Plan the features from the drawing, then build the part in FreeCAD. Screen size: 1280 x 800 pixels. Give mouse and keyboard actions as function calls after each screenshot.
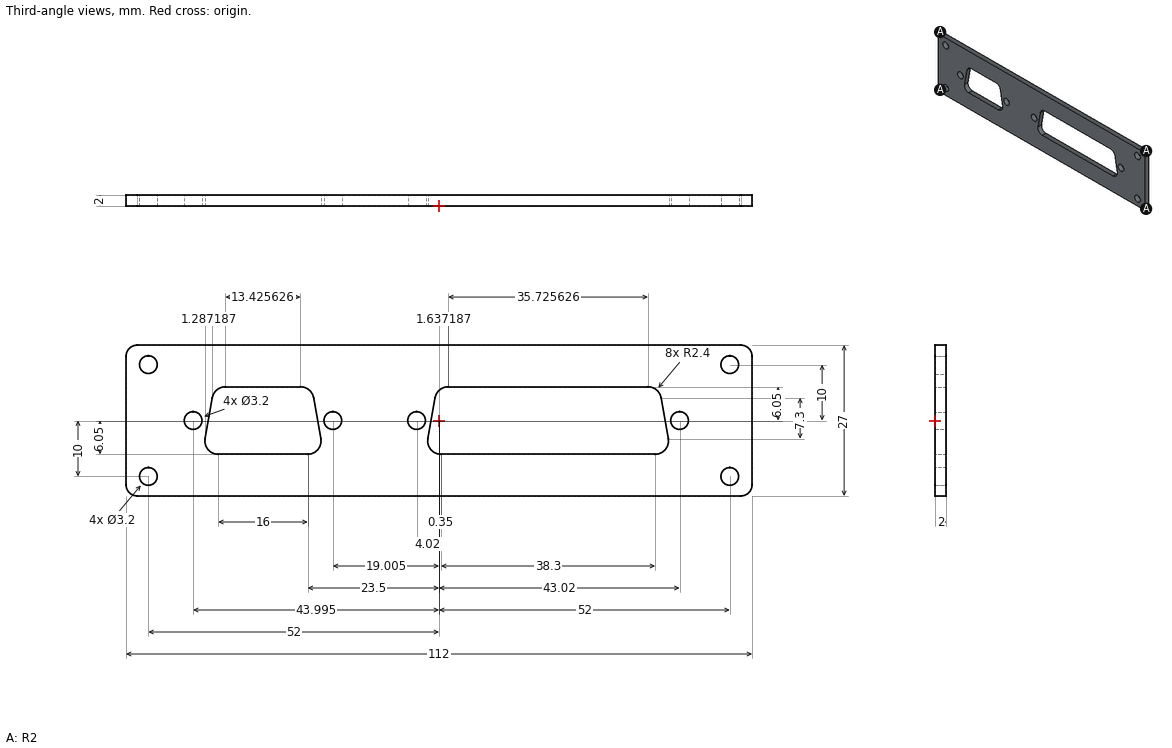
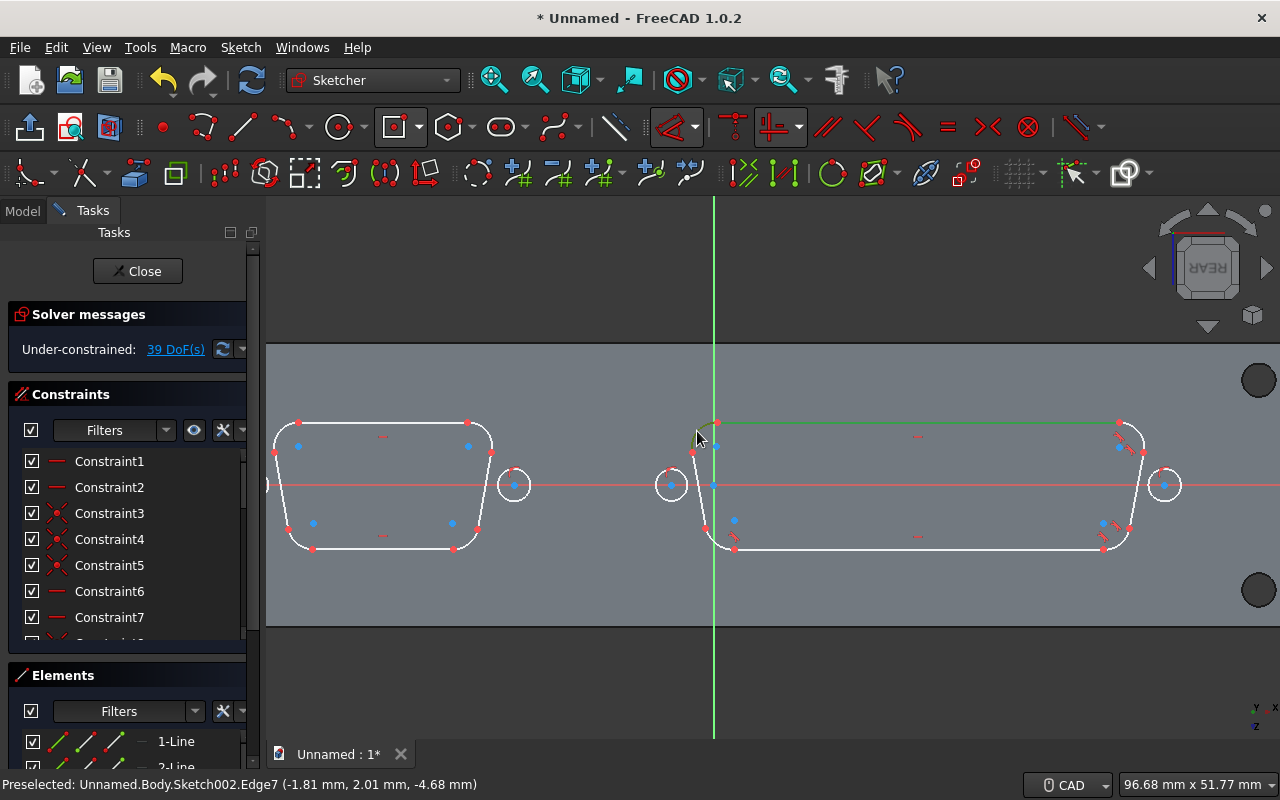
click(908, 128)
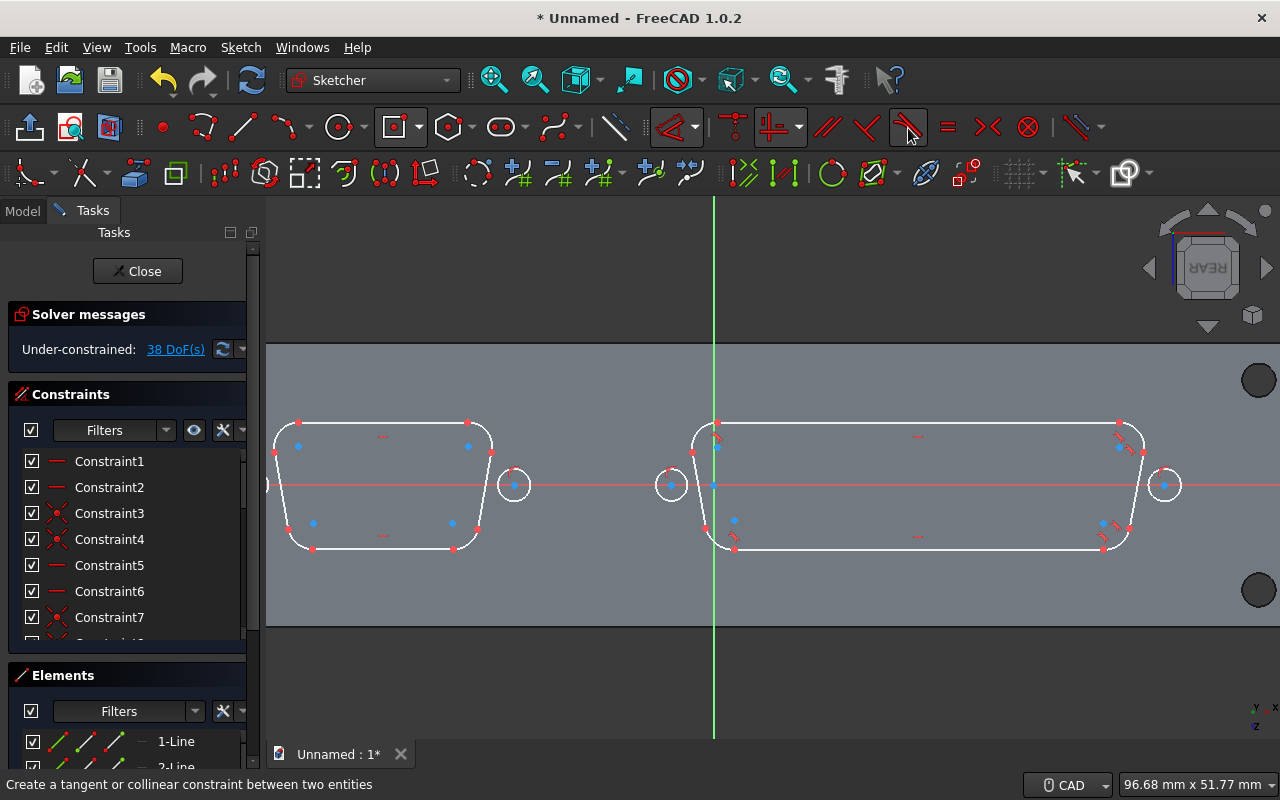
scroll(697, 475, up, 2)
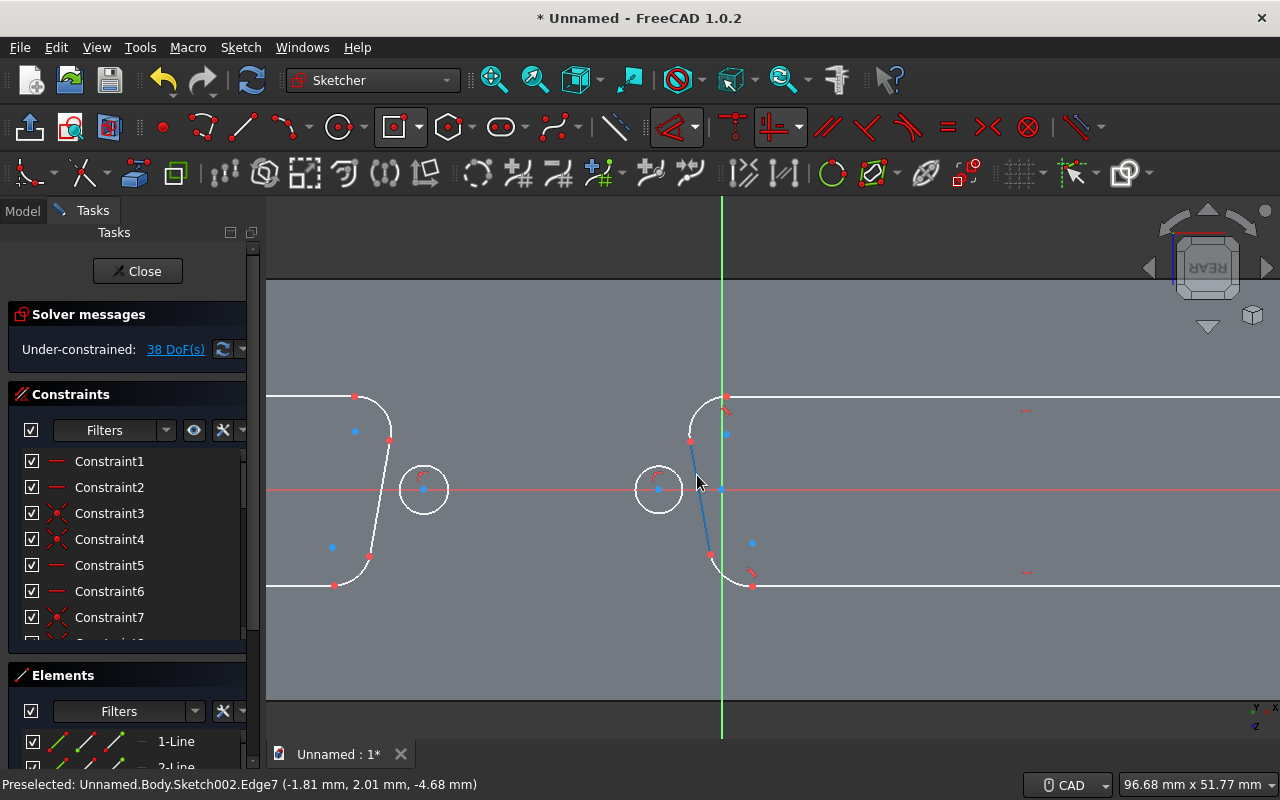
click(696, 475)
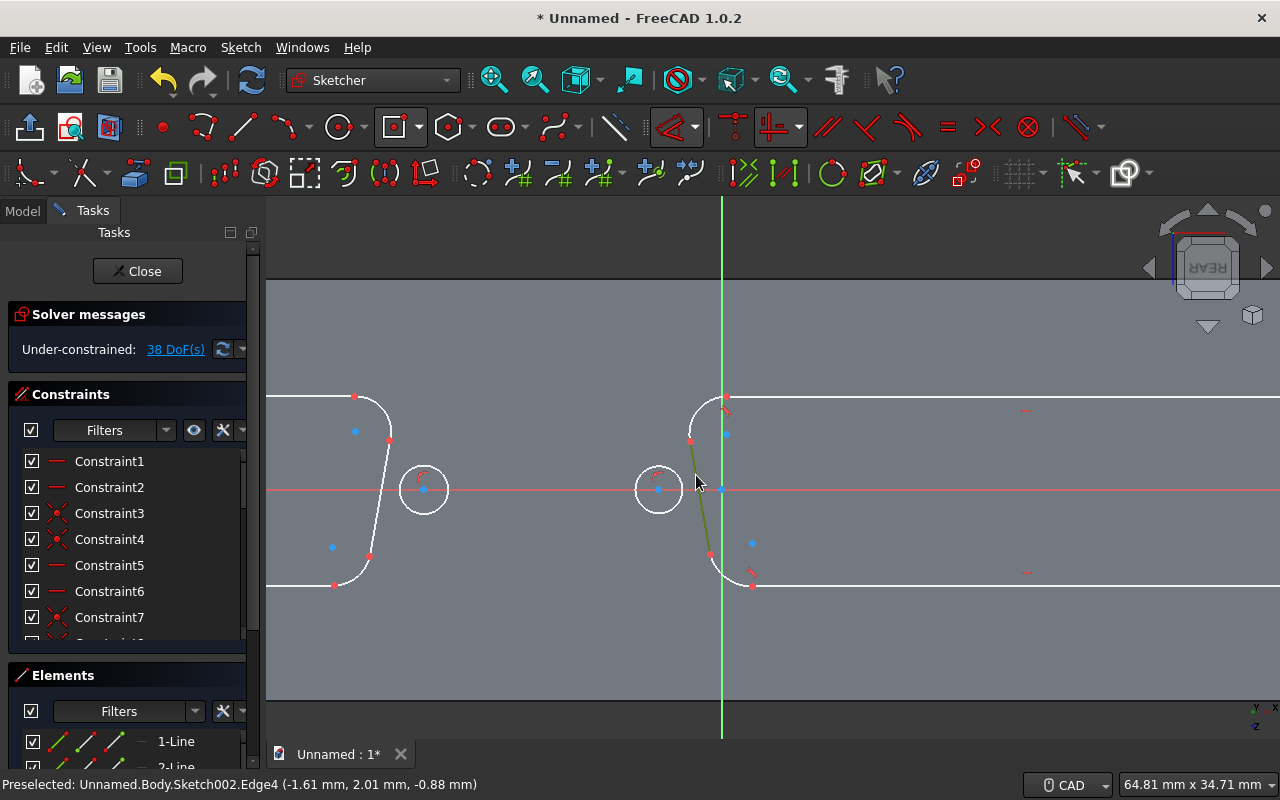
click(708, 402)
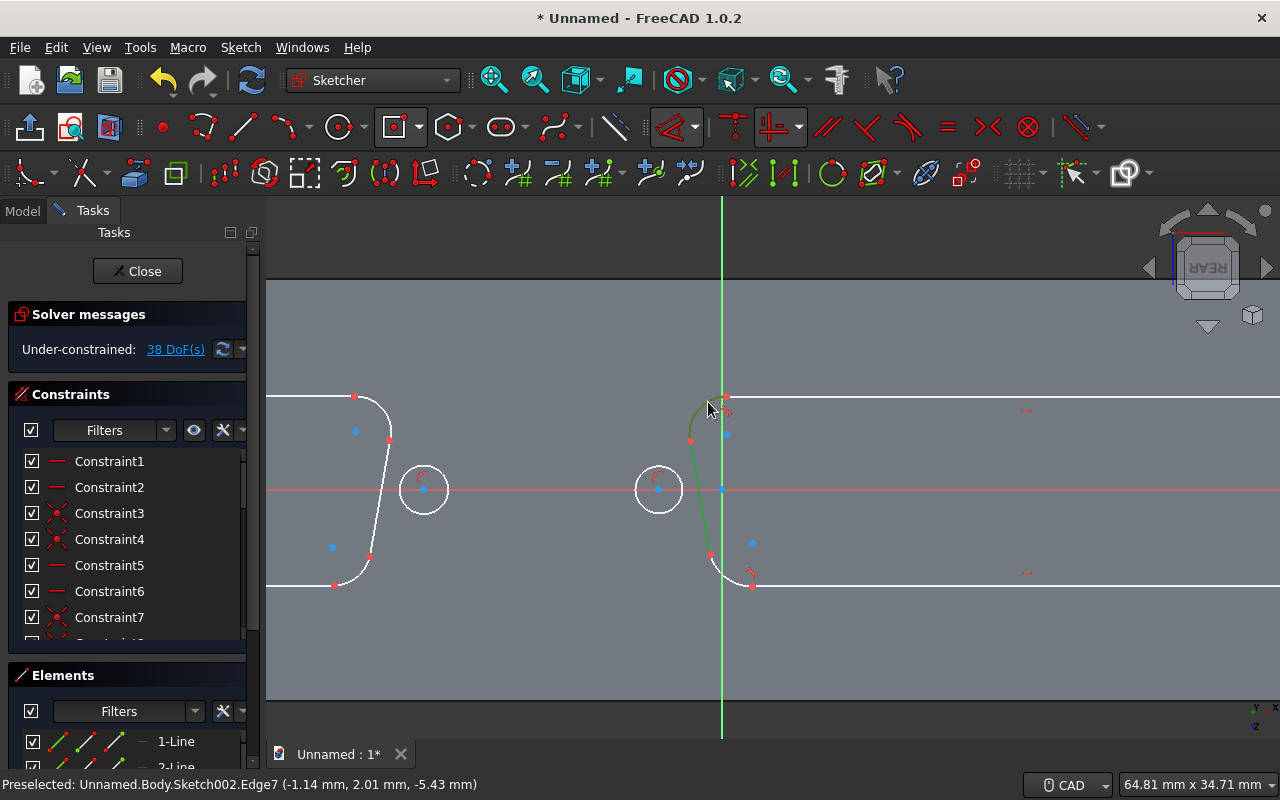
click(908, 128)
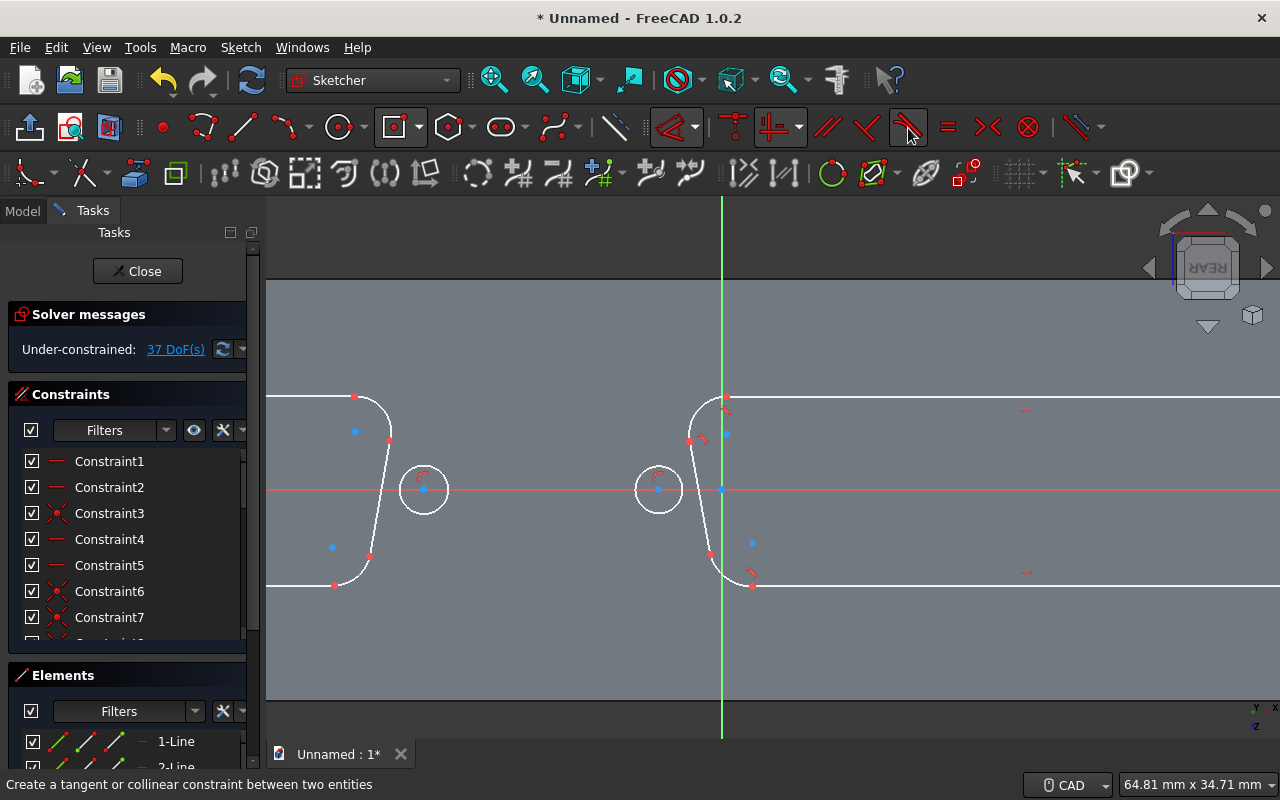
click(696, 475)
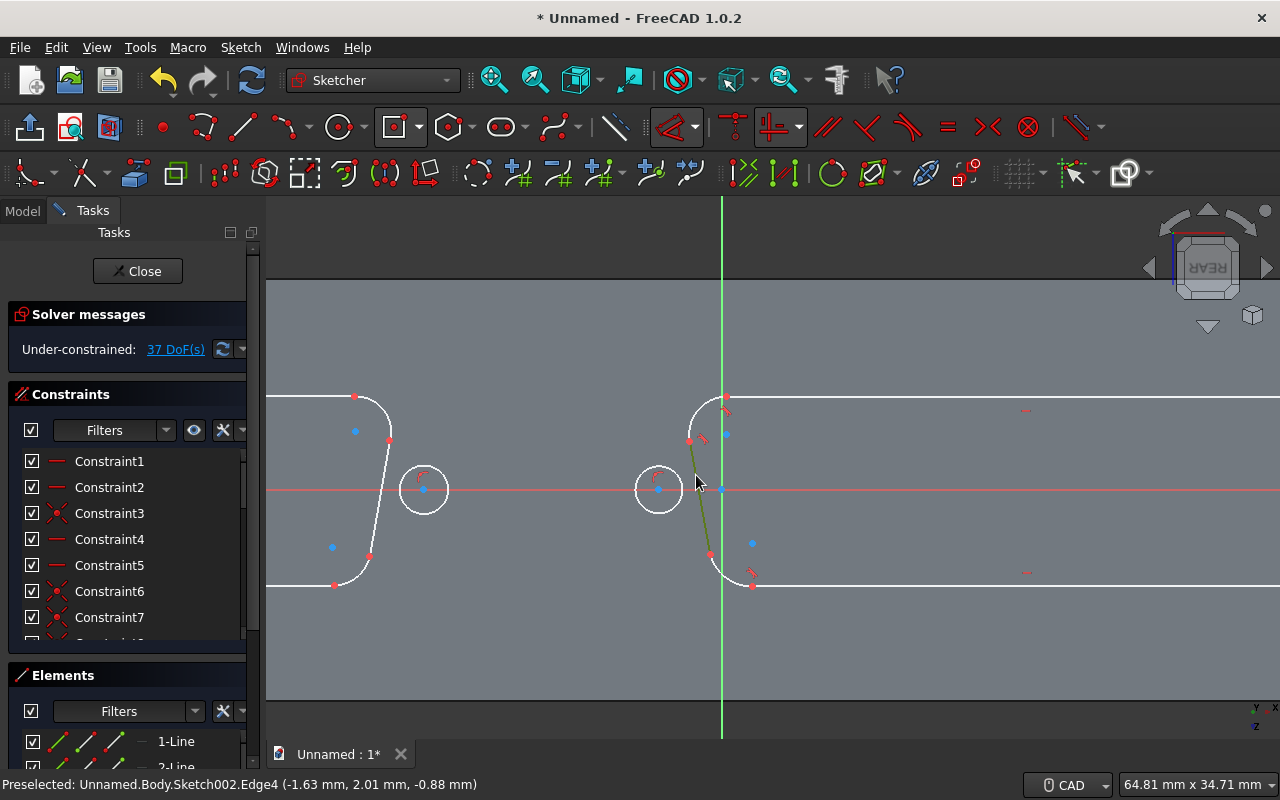
click(718, 569)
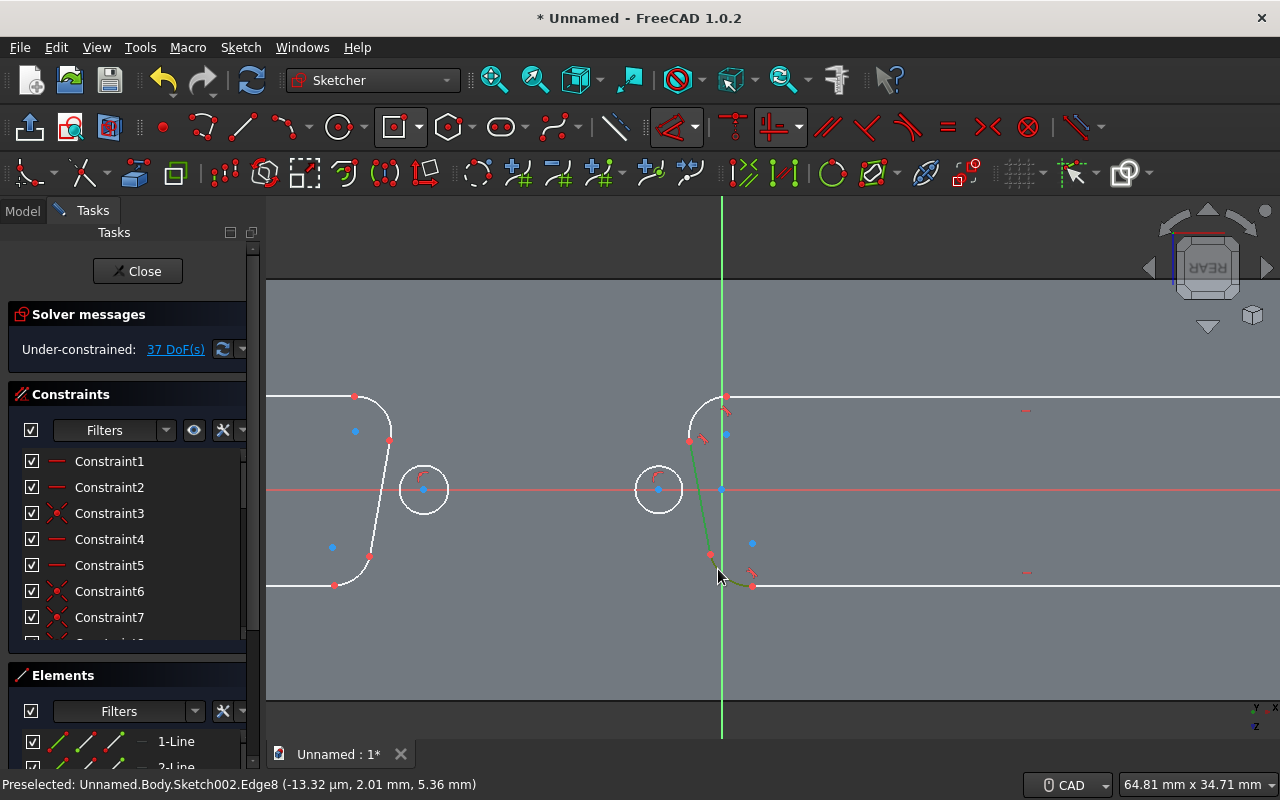
key(t)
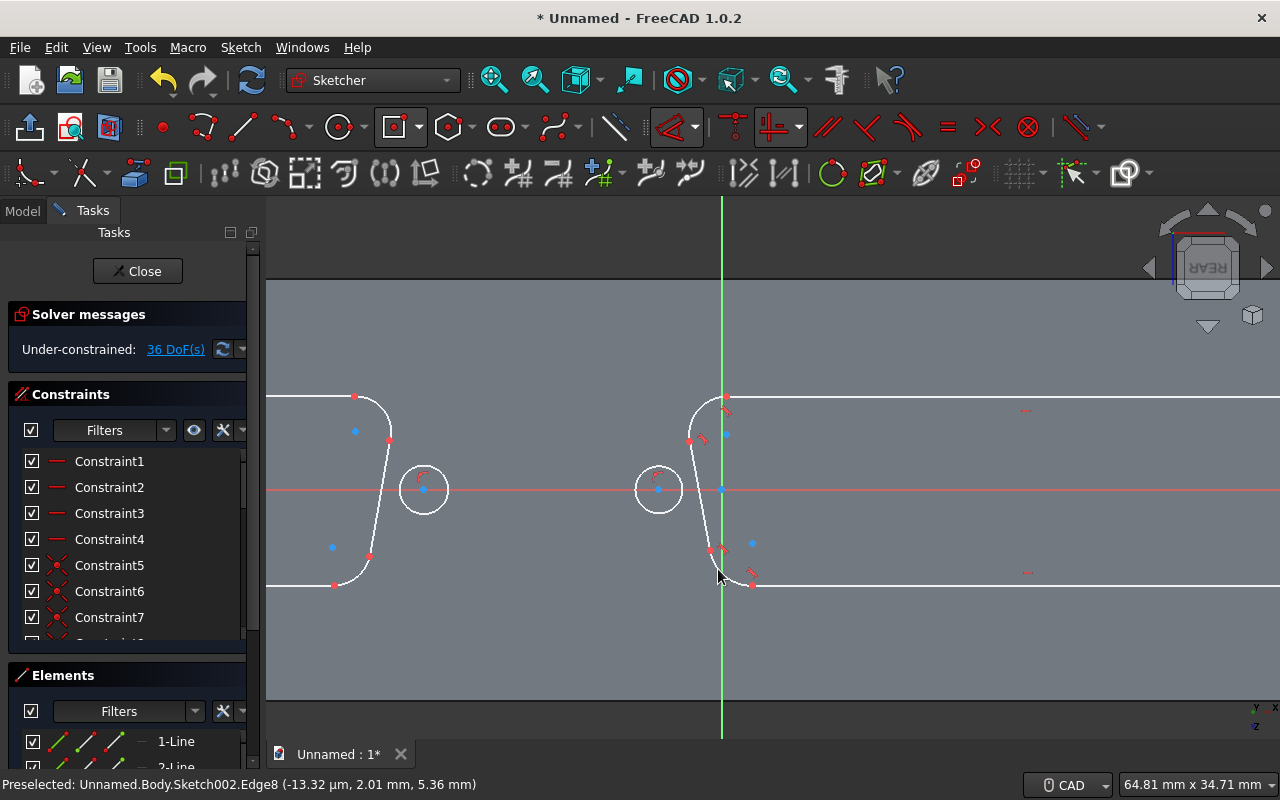
click(304, 396)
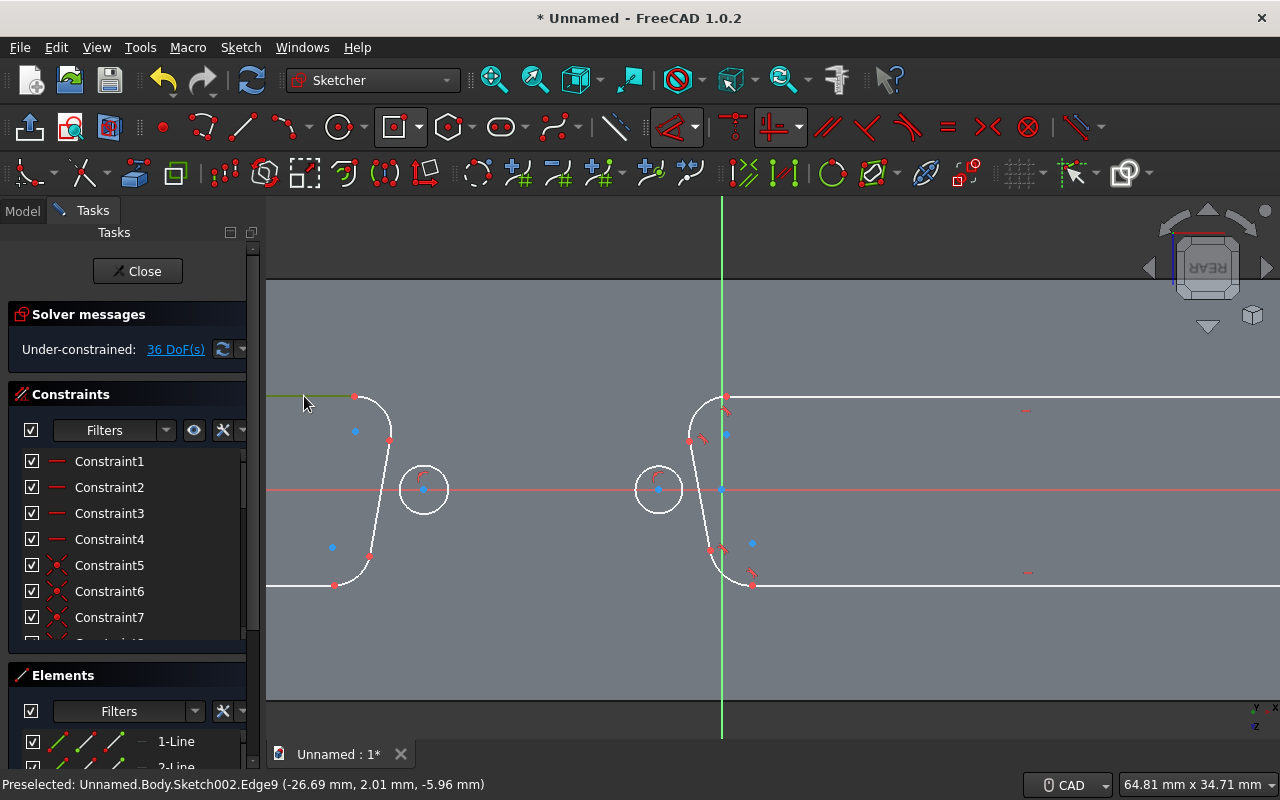
scroll(697, 449, down, 4)